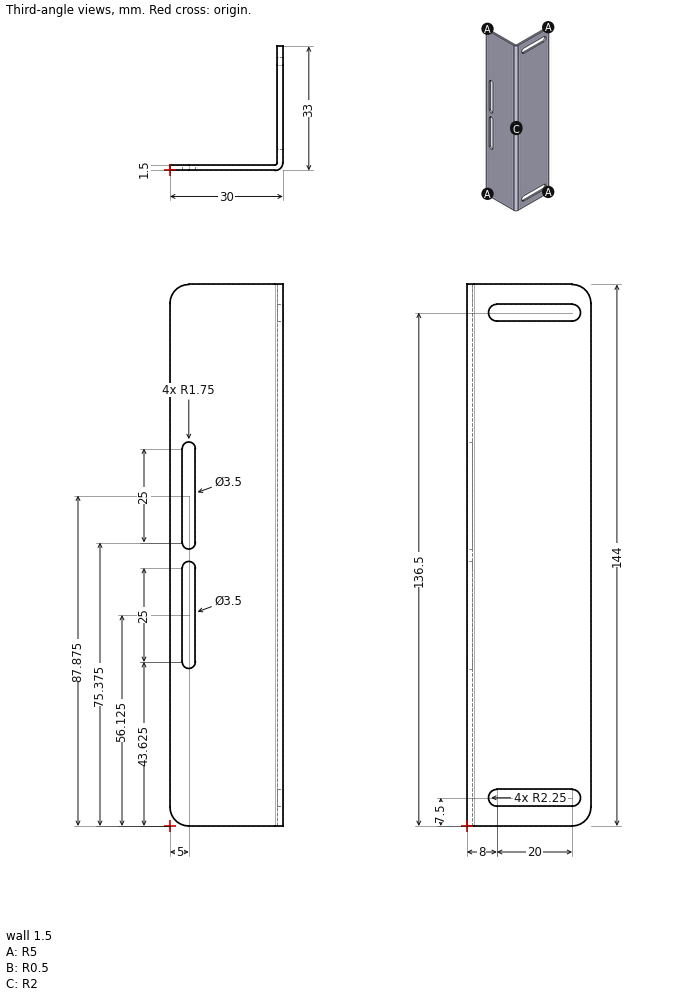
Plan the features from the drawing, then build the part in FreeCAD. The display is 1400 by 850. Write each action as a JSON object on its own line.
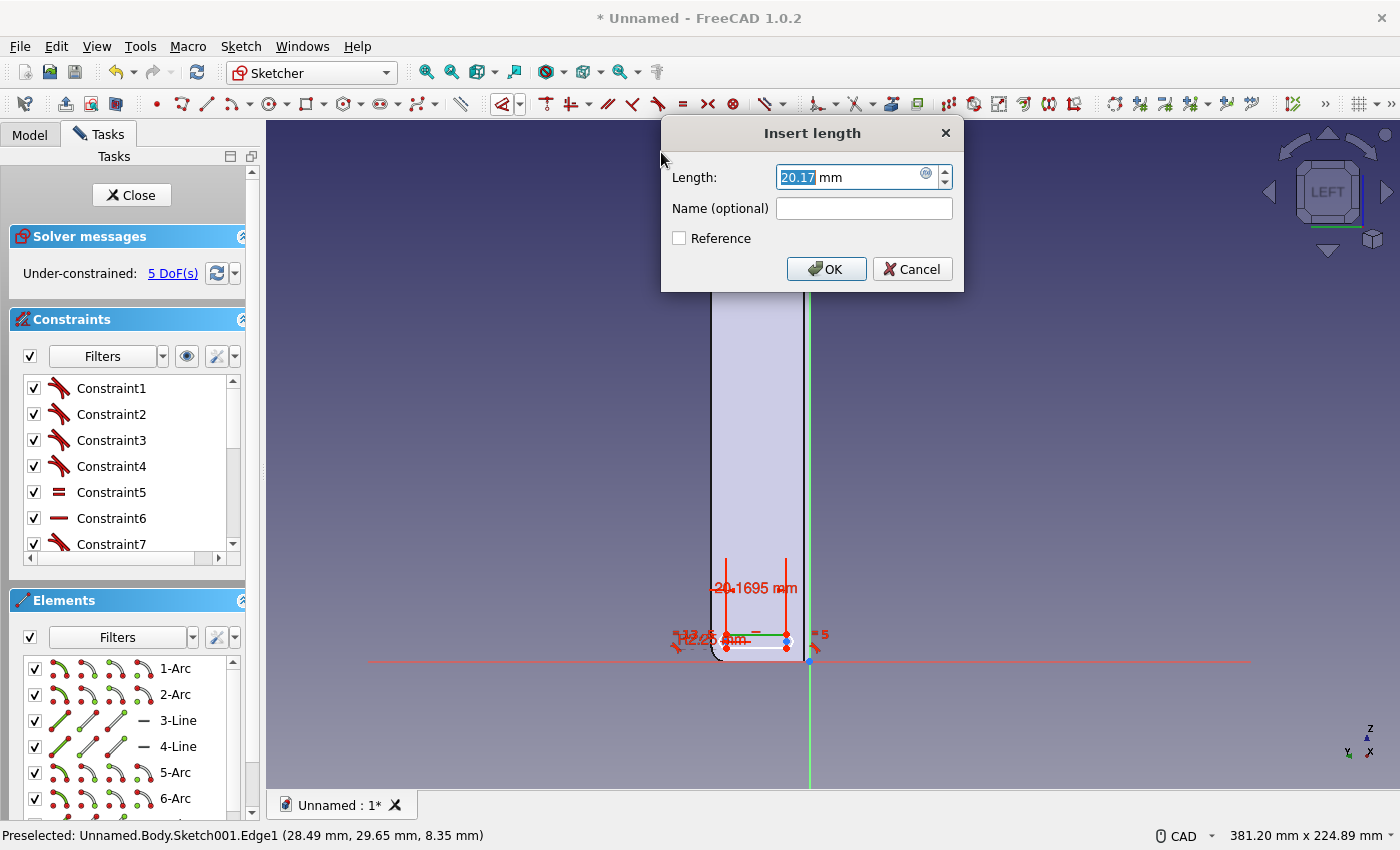
{"action": "type", "text": "20"}
{"action": "key", "text": "Return"}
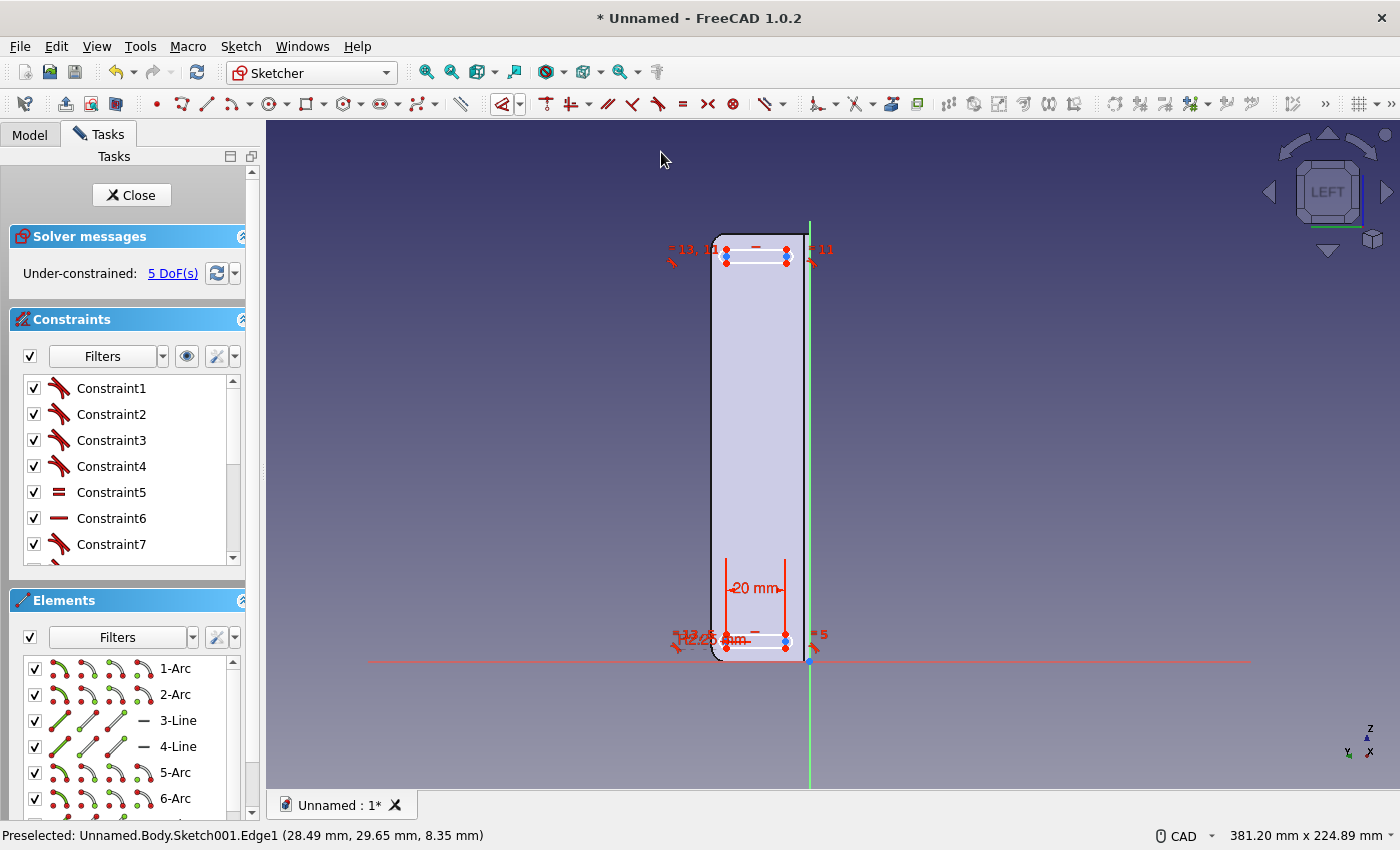
{"action": "left_click", "coordinate": [744, 250]}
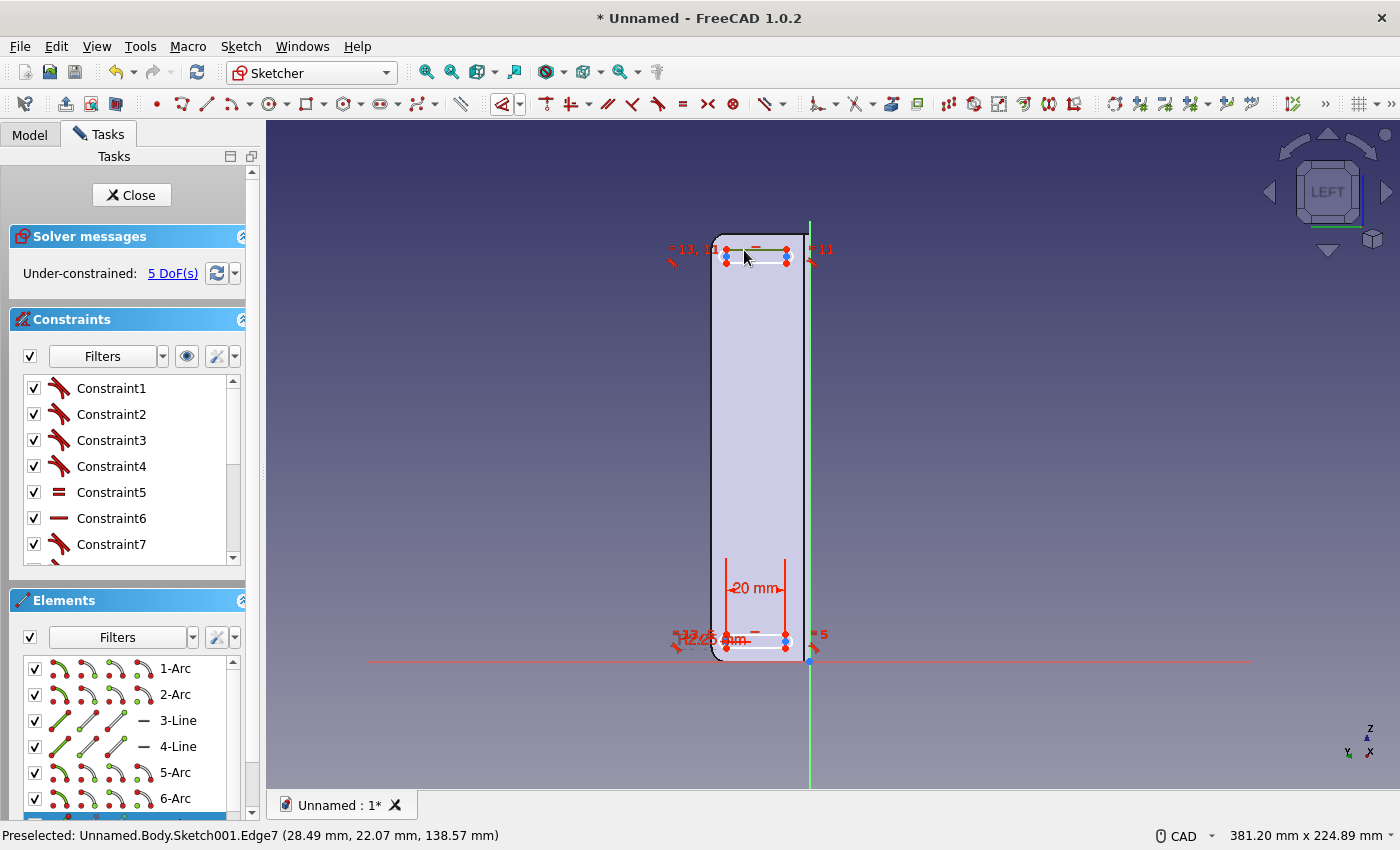
{"action": "key", "text": "l"}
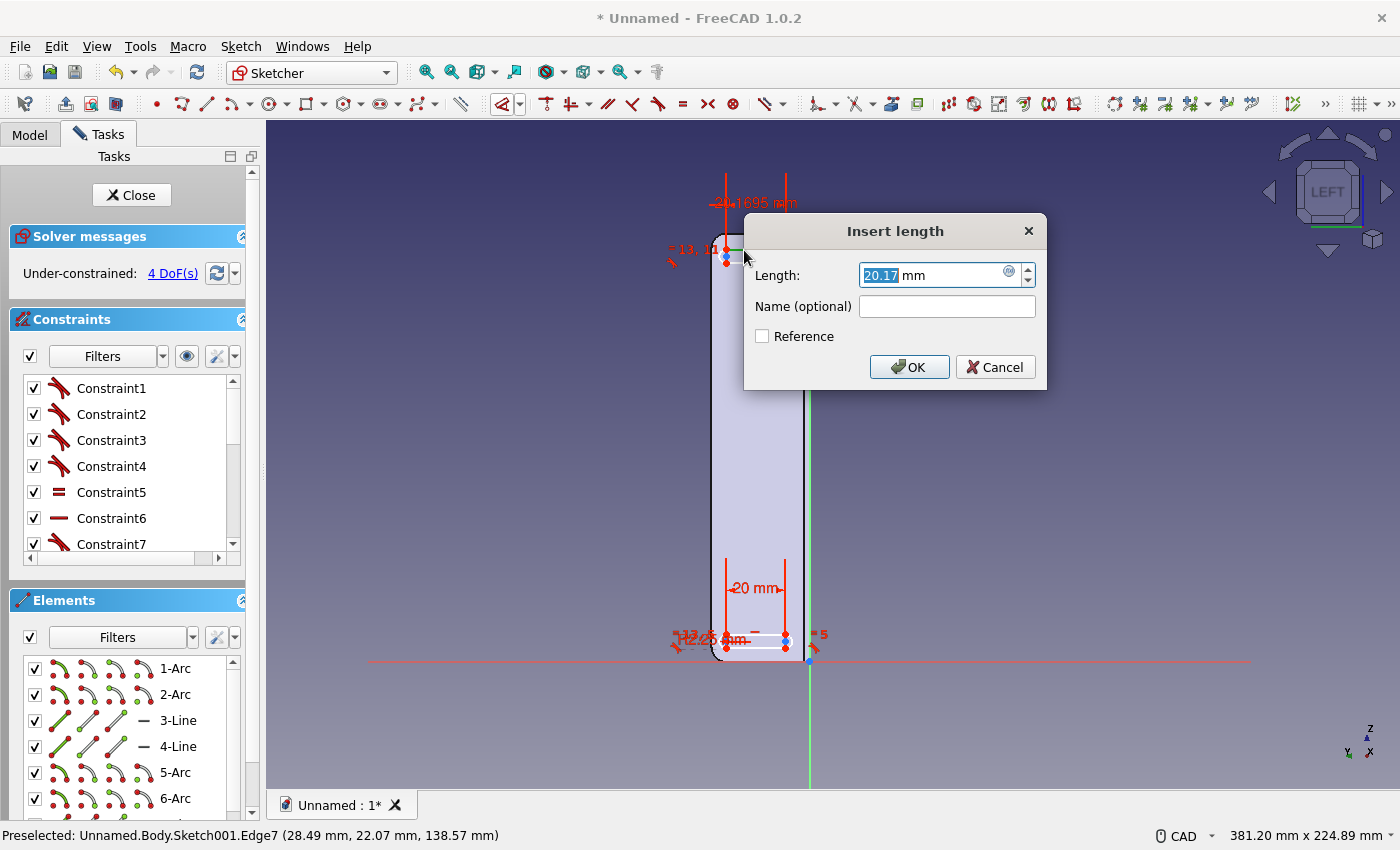
{"action": "type", "text": "20"}
{"action": "key", "text": "Return"}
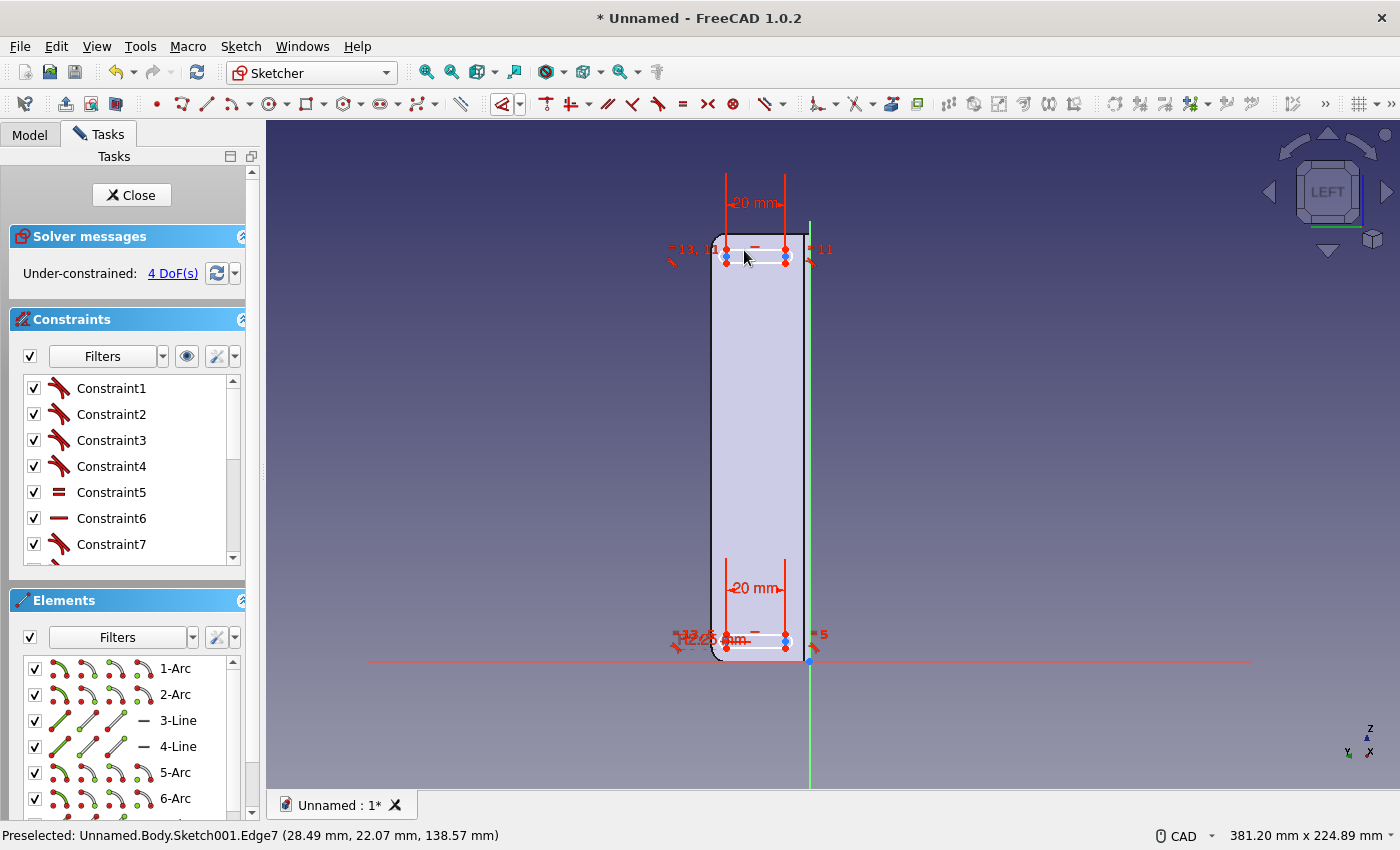
{"action": "scroll", "coordinate": [785, 648], "scroll_direction": "up", "scroll_amount": 4}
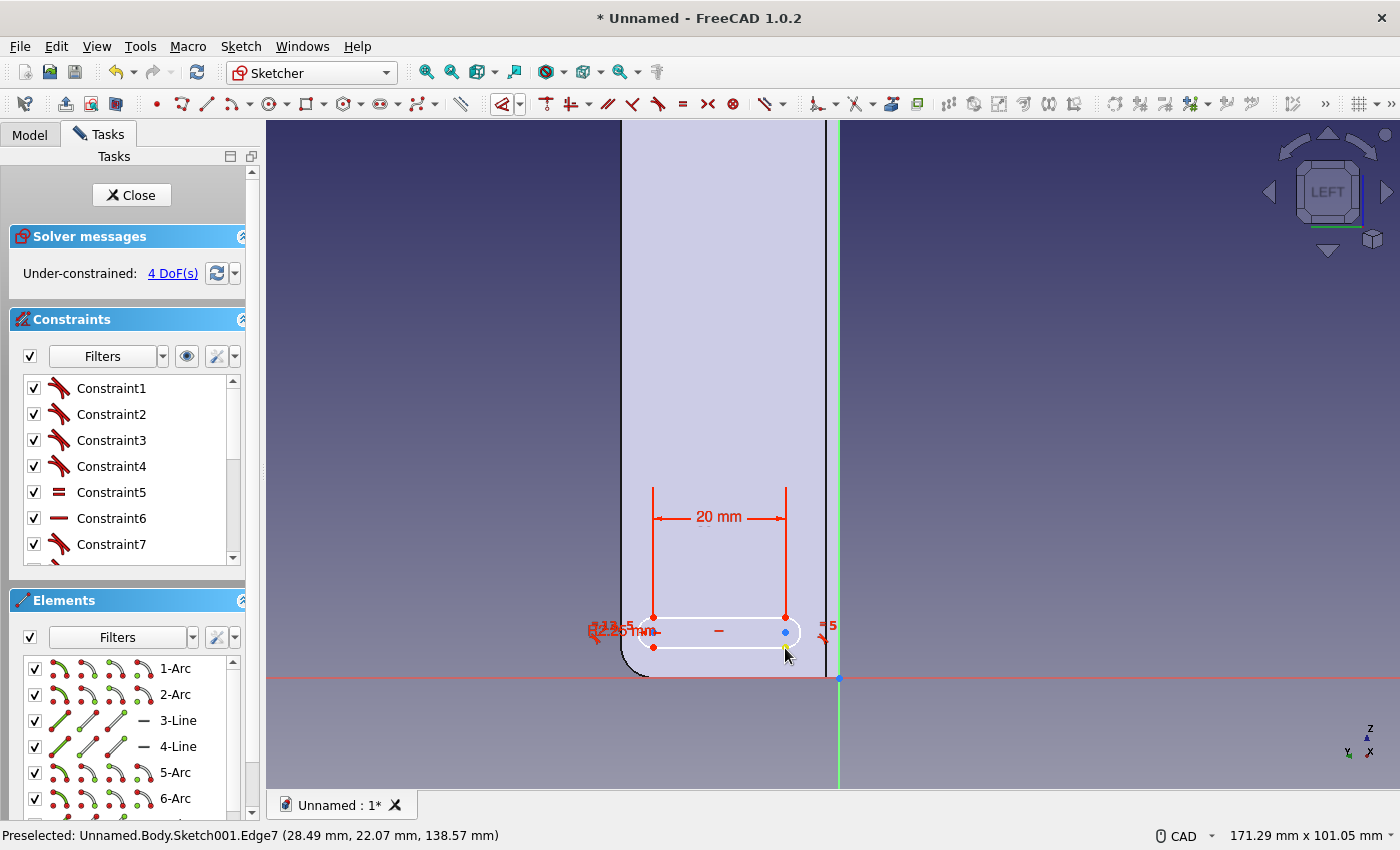
{"action": "left_click", "coordinate": [786, 648]}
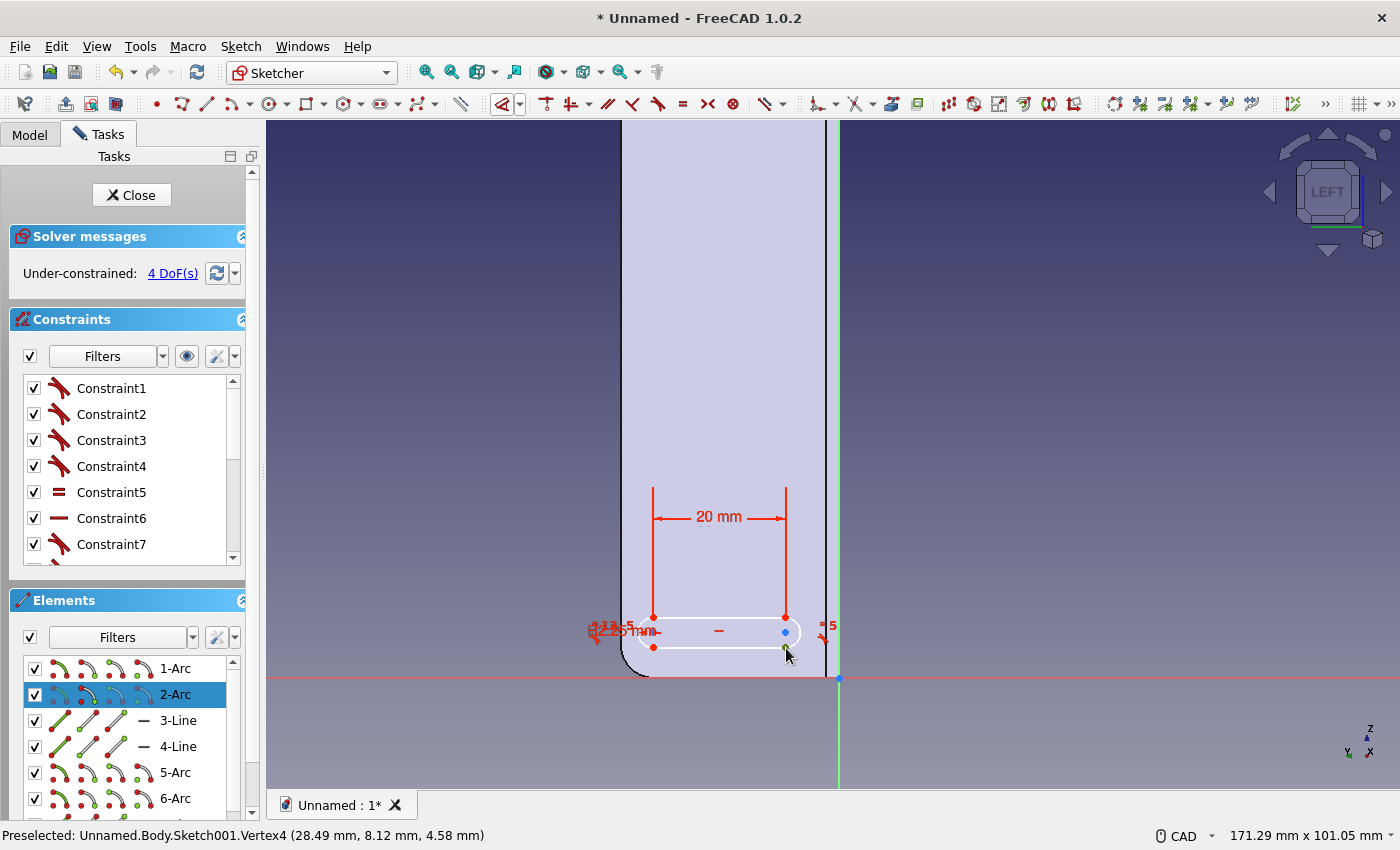
{"action": "left_click", "coordinate": [520, 104]}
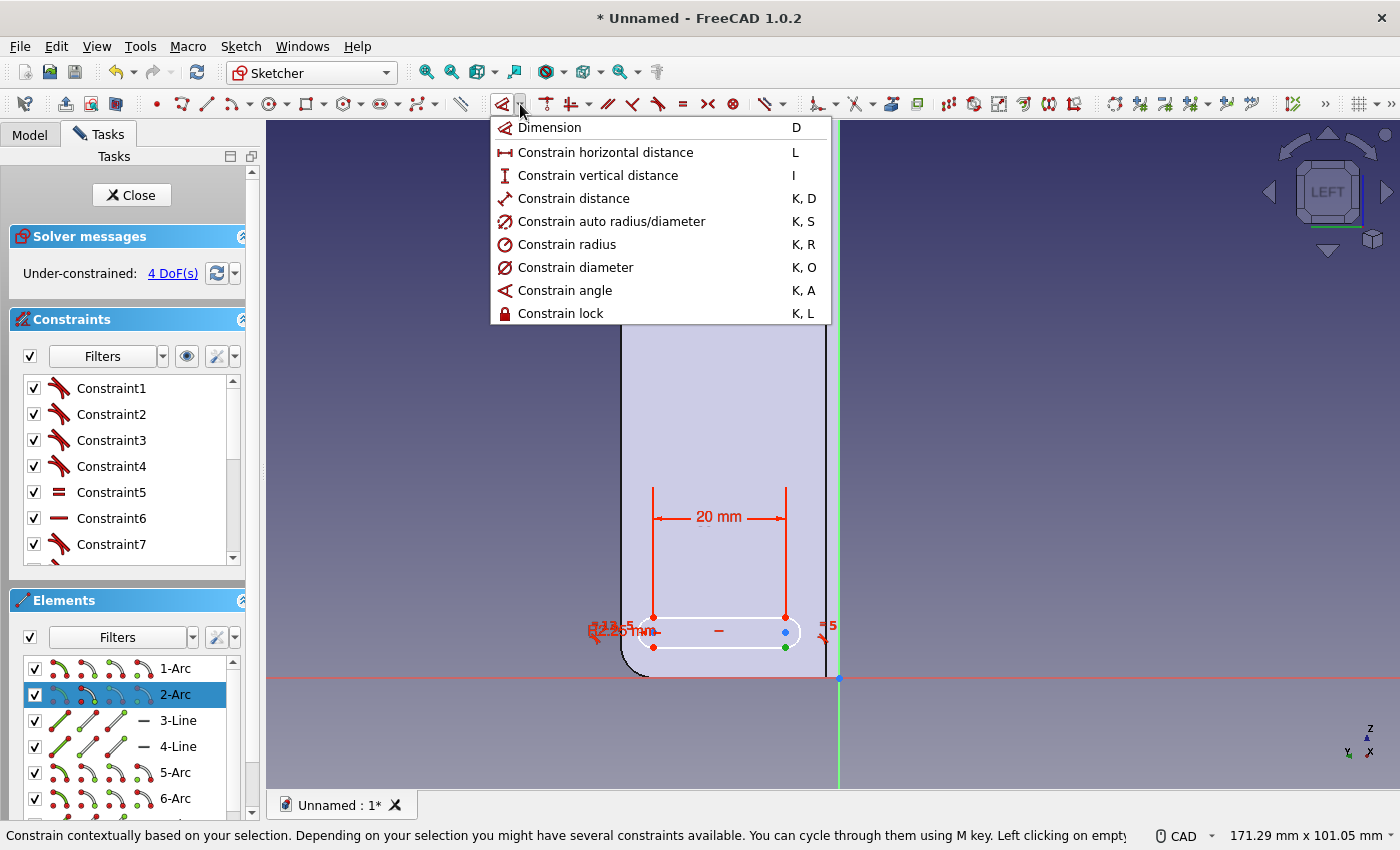
{"action": "left_click", "coordinate": [661, 152]}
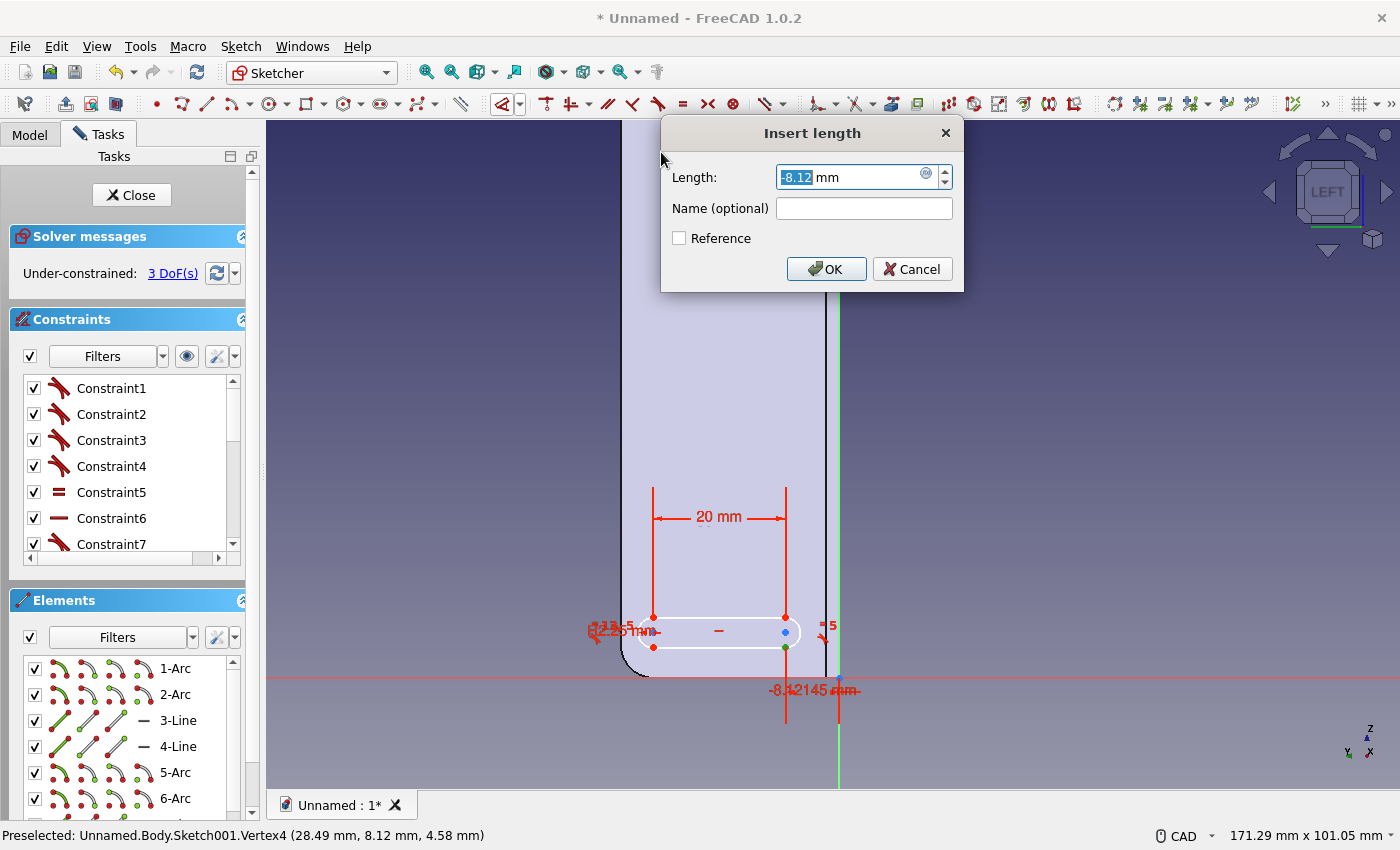
{"action": "type", "text": "-8"}
{"action": "key", "text": "Return"}